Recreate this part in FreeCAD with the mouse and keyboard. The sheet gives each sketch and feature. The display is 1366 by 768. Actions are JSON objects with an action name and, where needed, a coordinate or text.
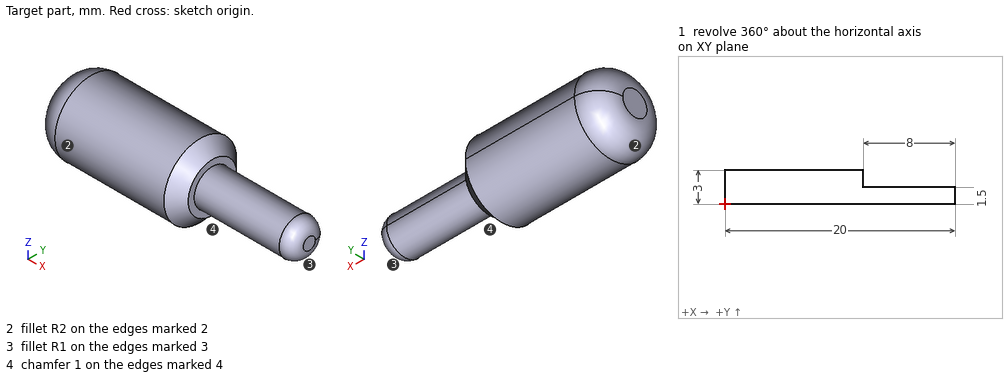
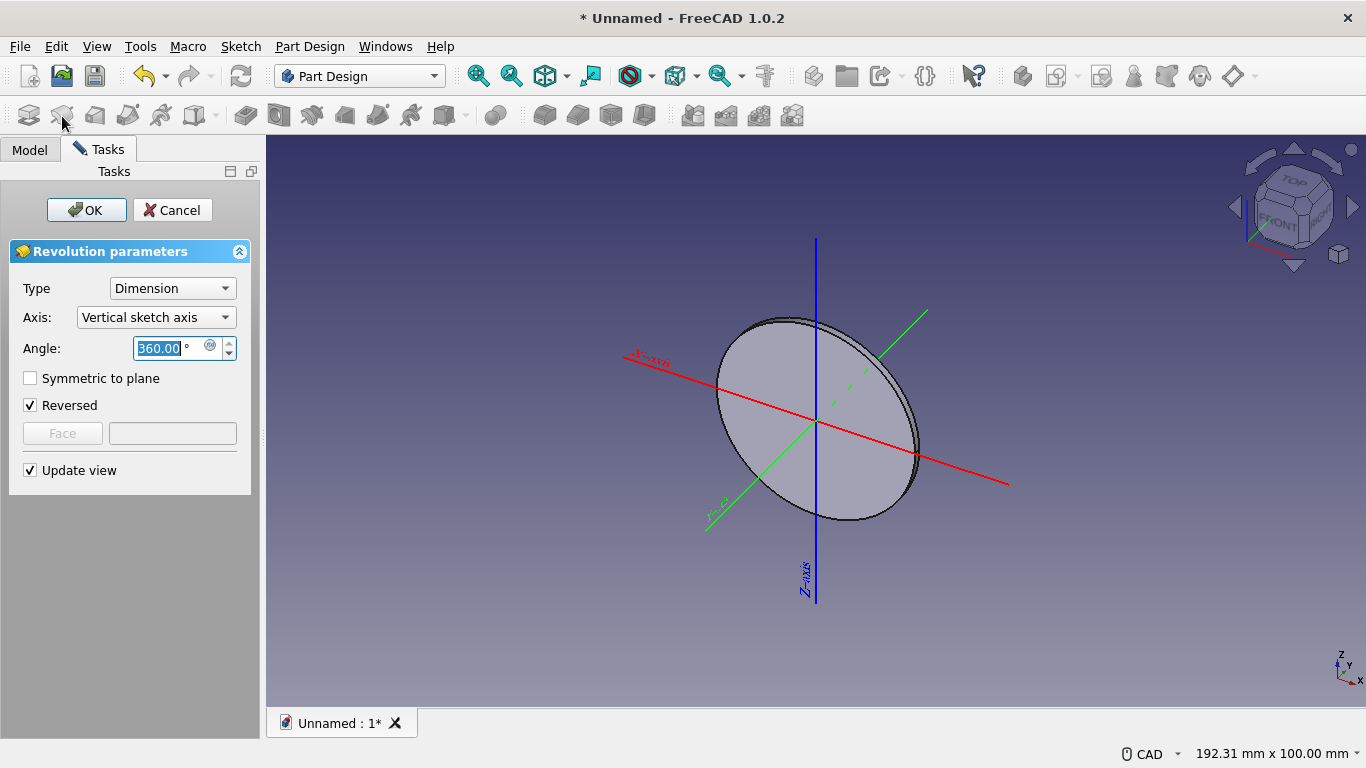
{"action": "left_click", "coordinate": [157, 318]}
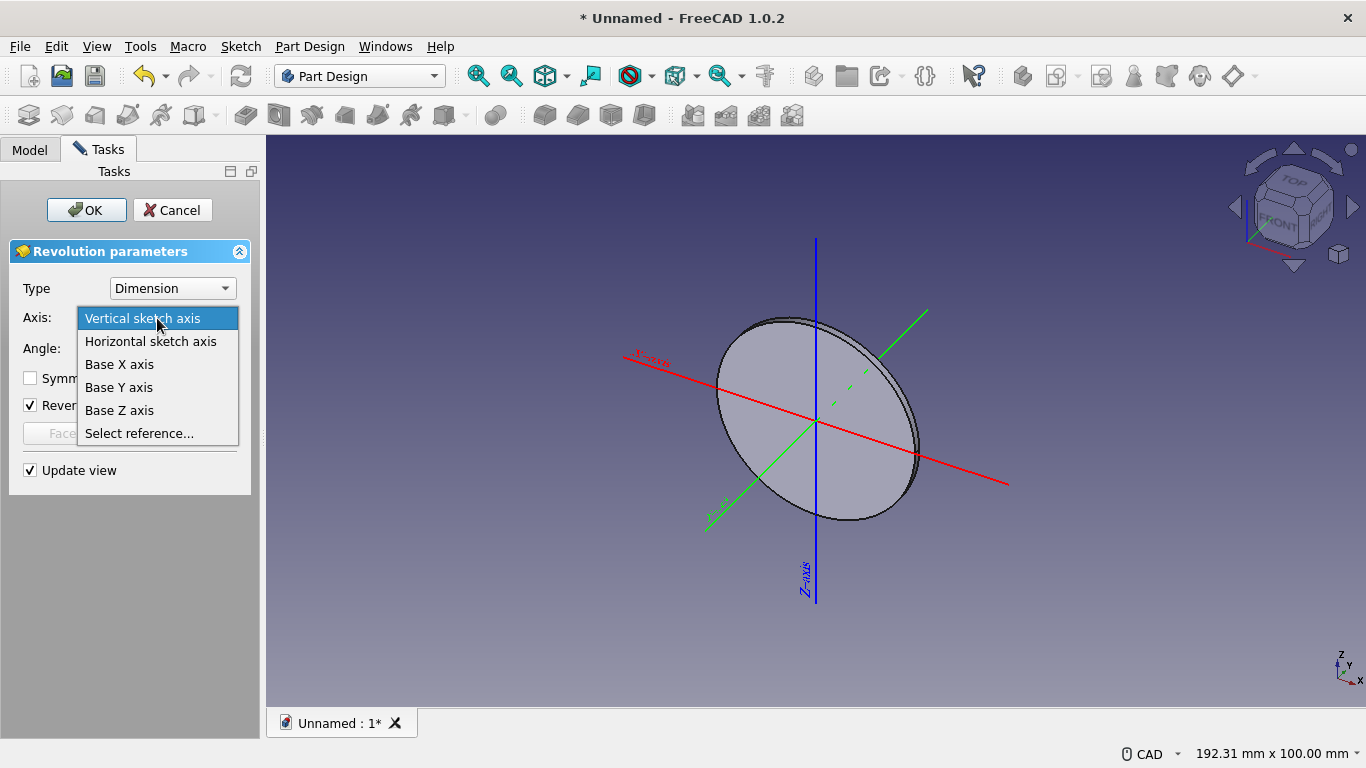
{"action": "left_click", "coordinate": [156, 342]}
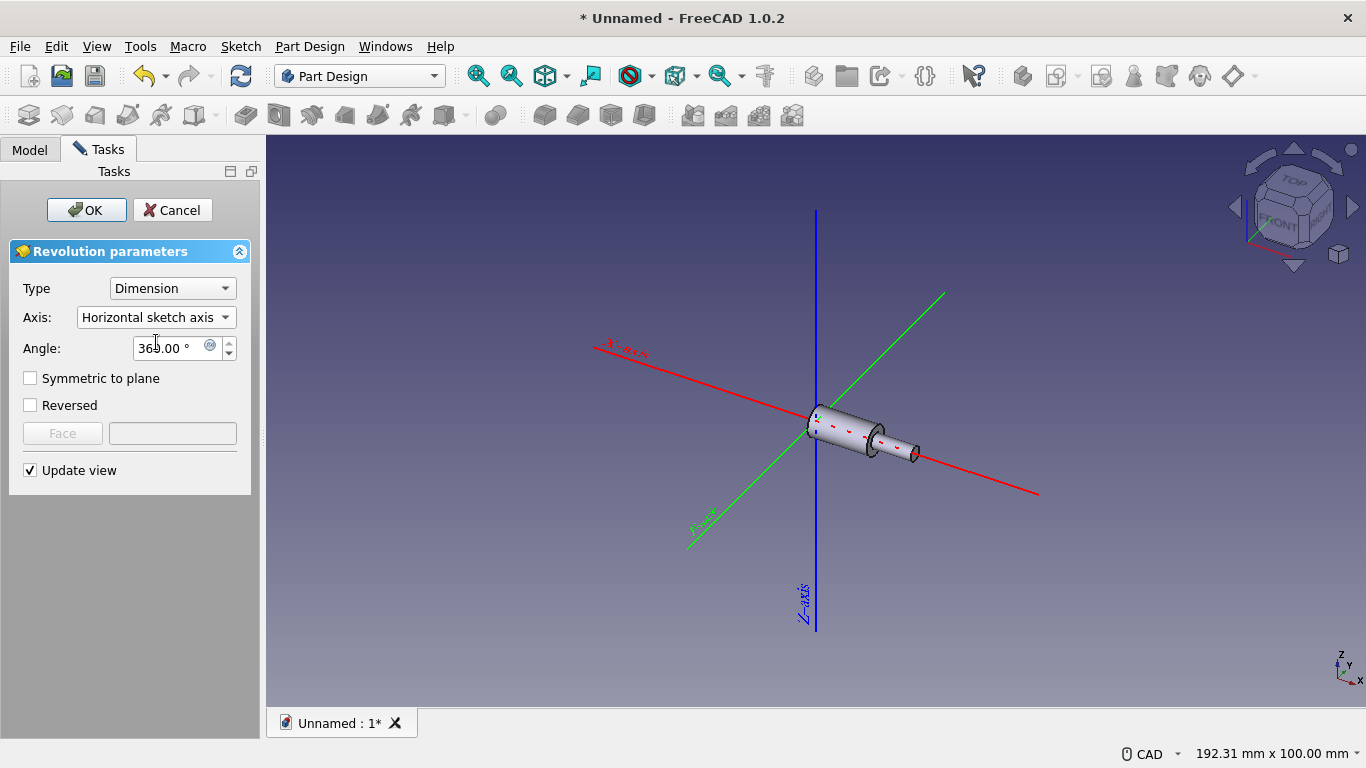
{"action": "left_click", "coordinate": [87, 210]}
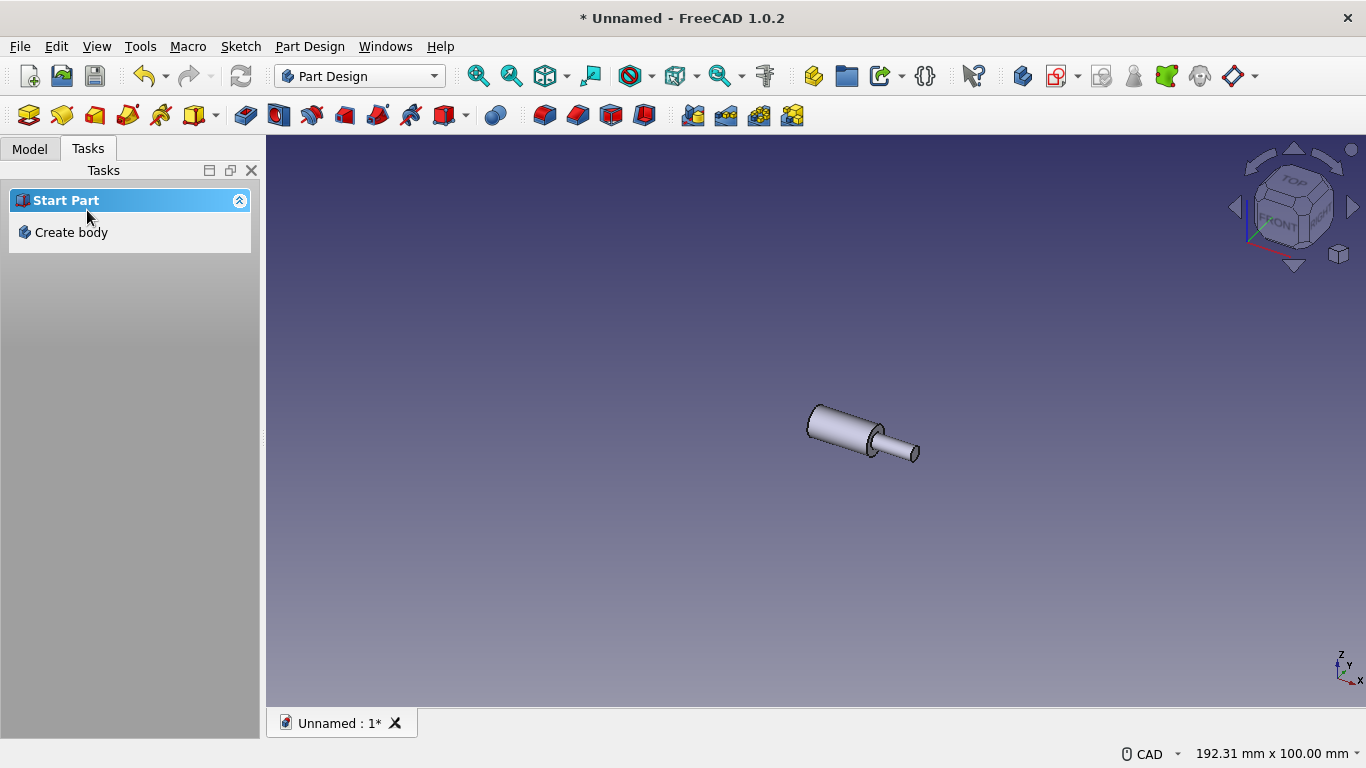
{"action": "left_click", "coordinate": [479, 76]}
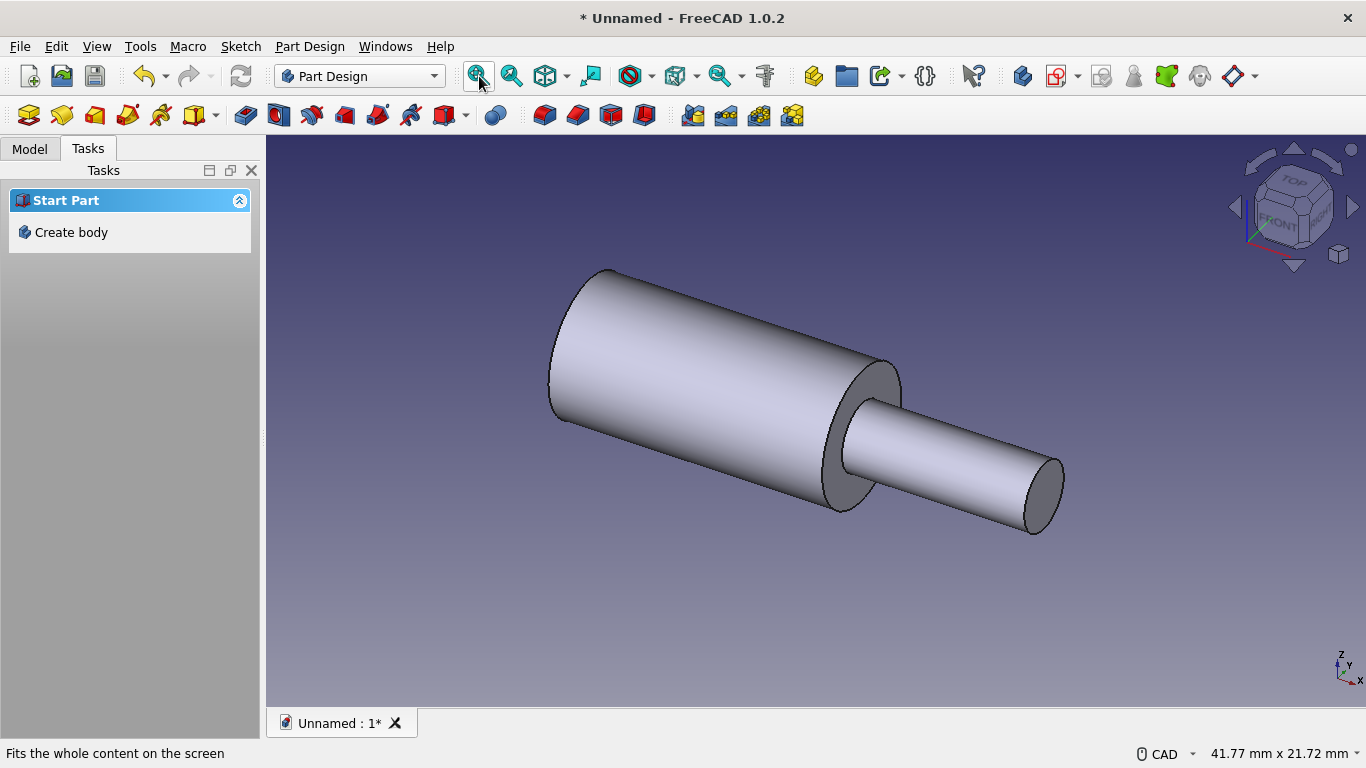
{"action": "left_click", "coordinate": [600, 271]}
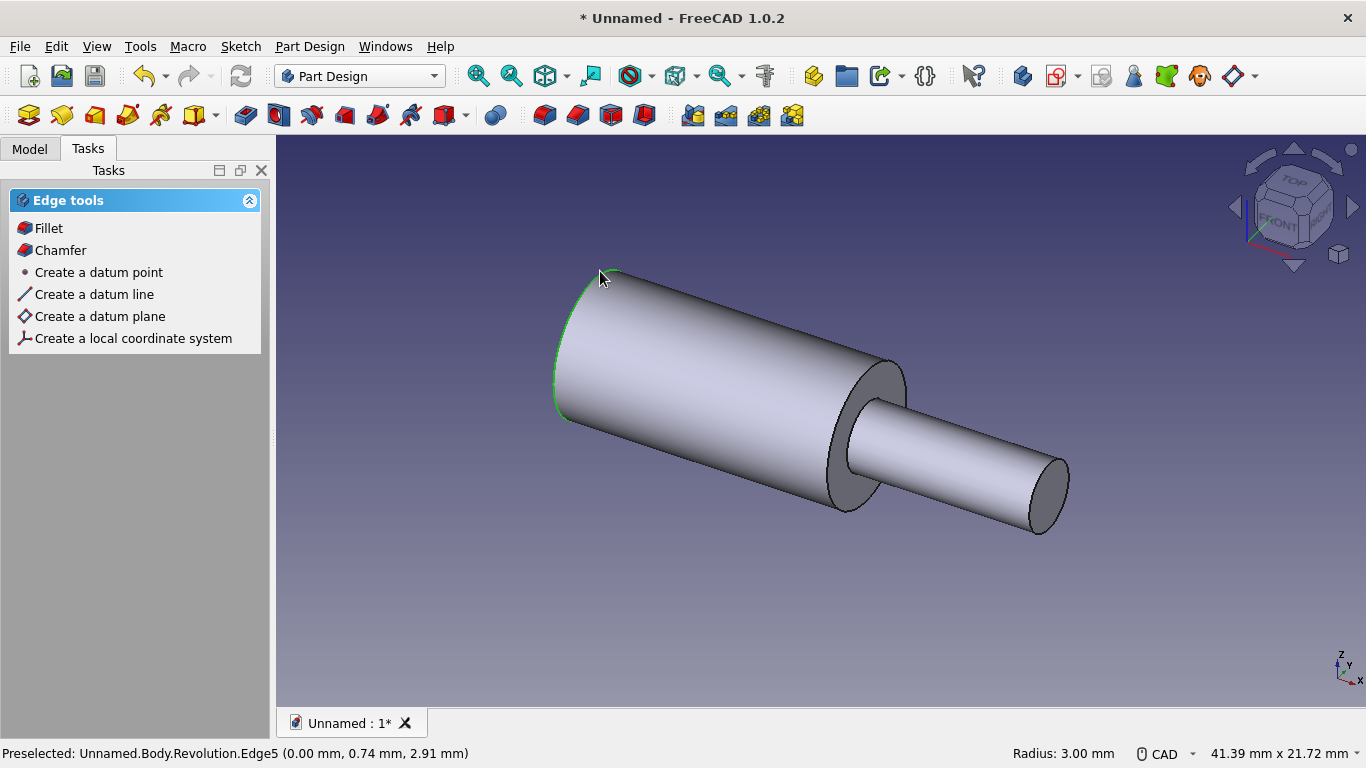
{"action": "left_click", "coordinate": [545, 116]}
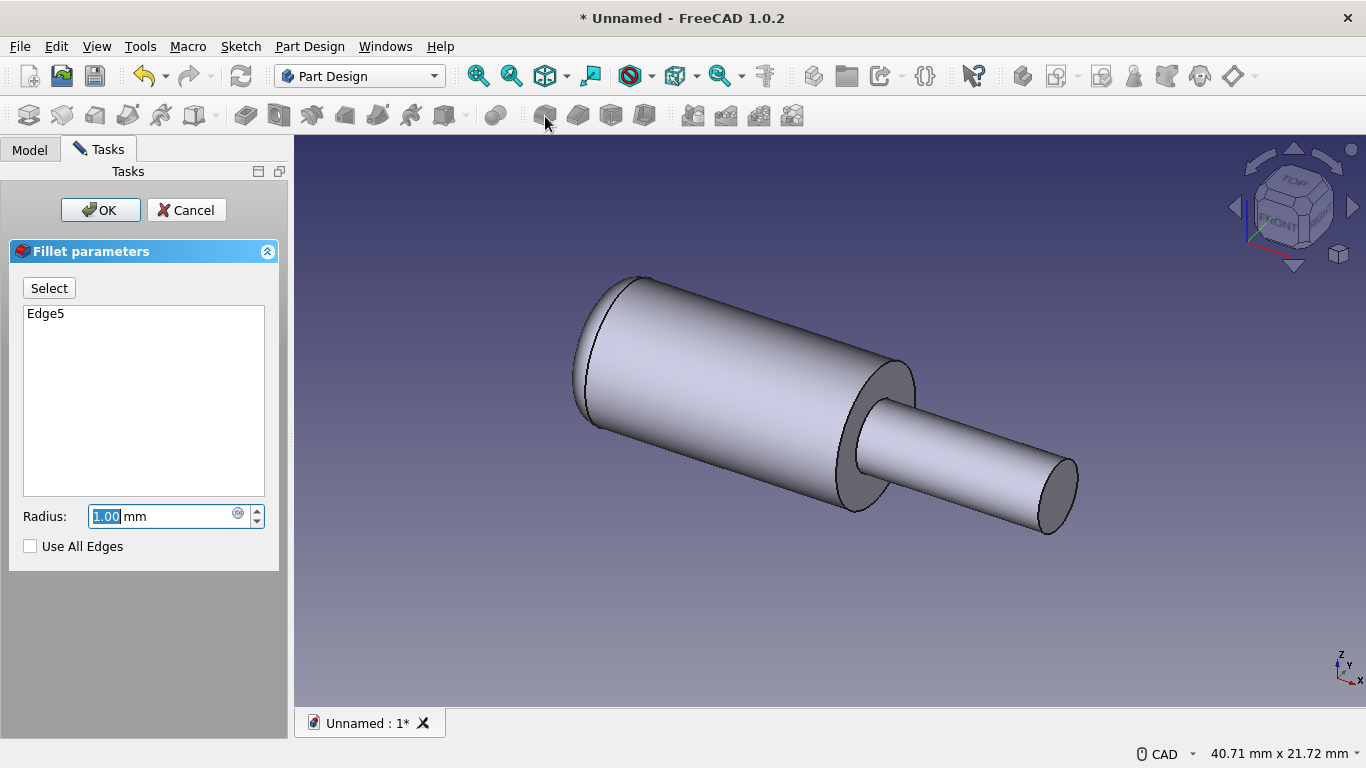
{"action": "type", "text": "2"}
{"action": "key", "text": "Tab"}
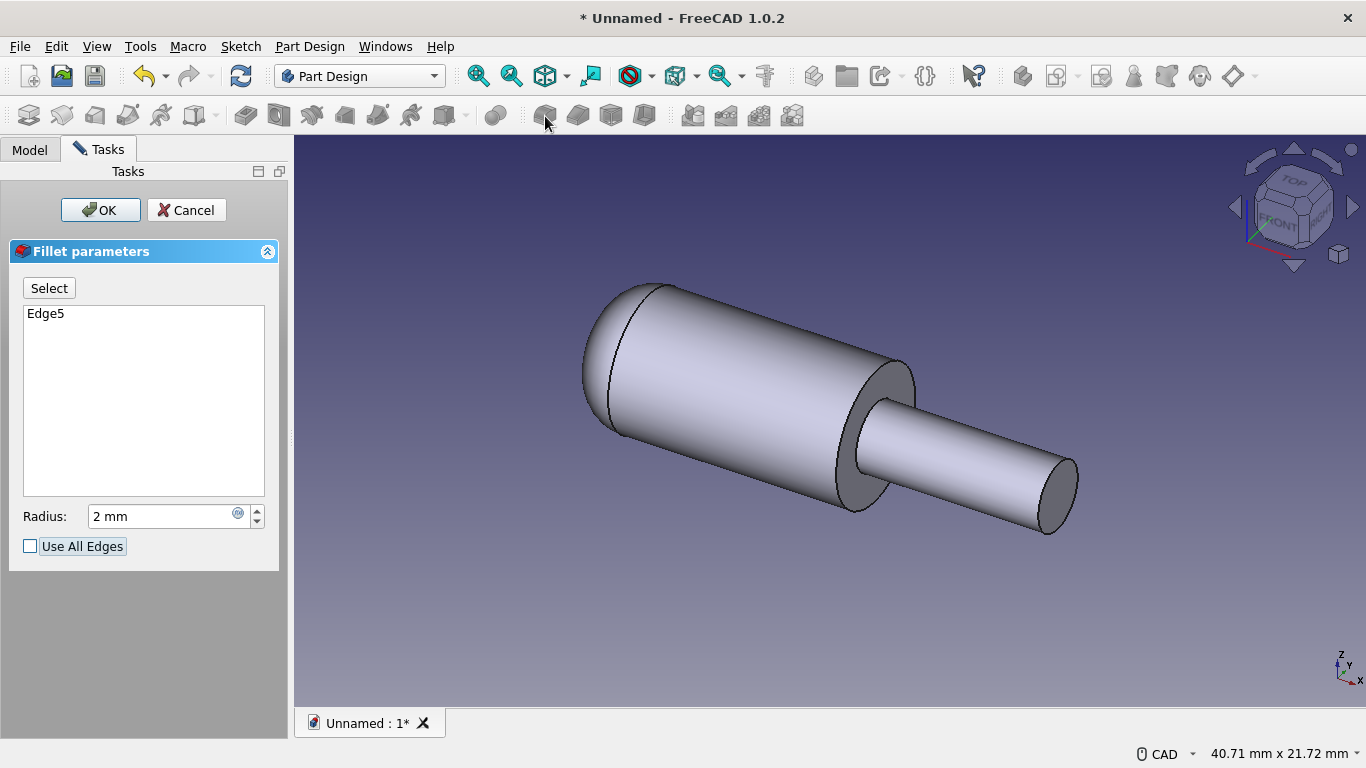
{"action": "left_click", "coordinate": [101, 210]}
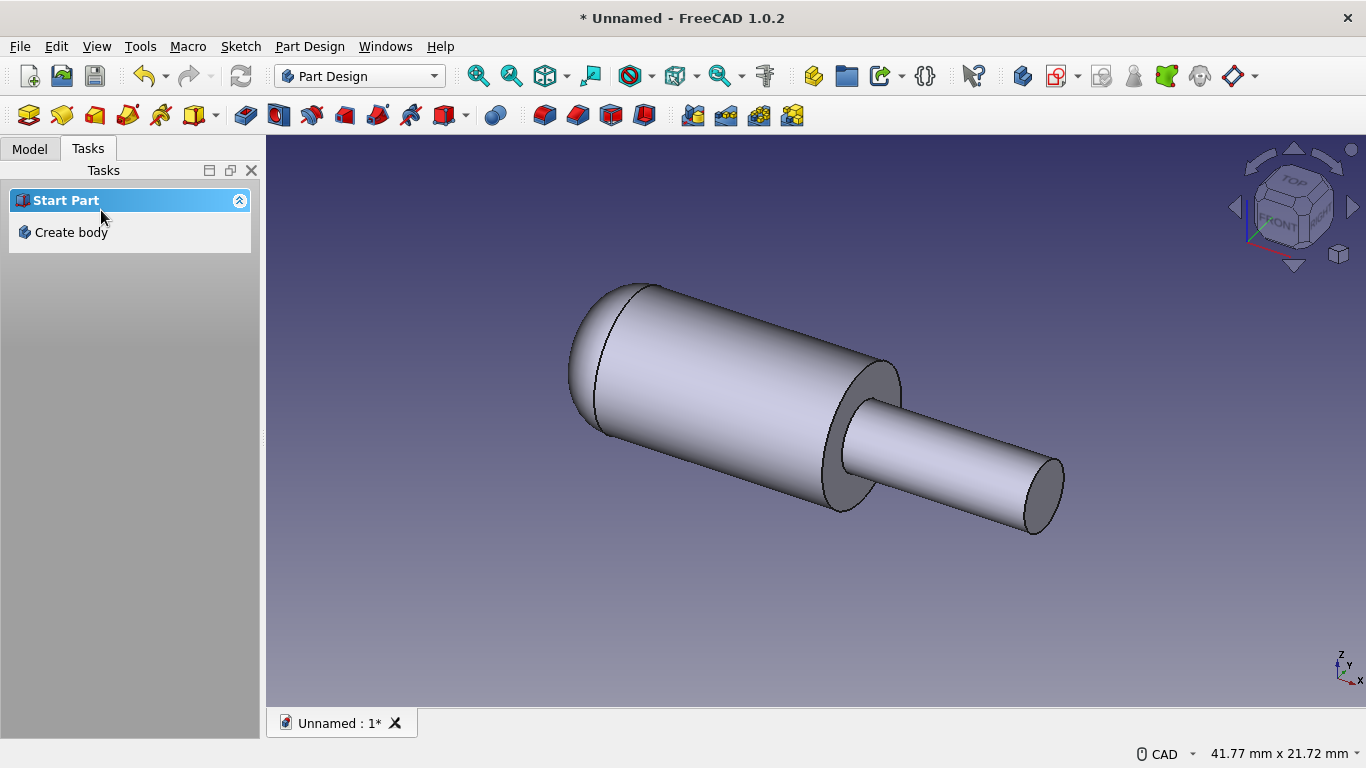
{"action": "left_click", "coordinate": [1024, 515]}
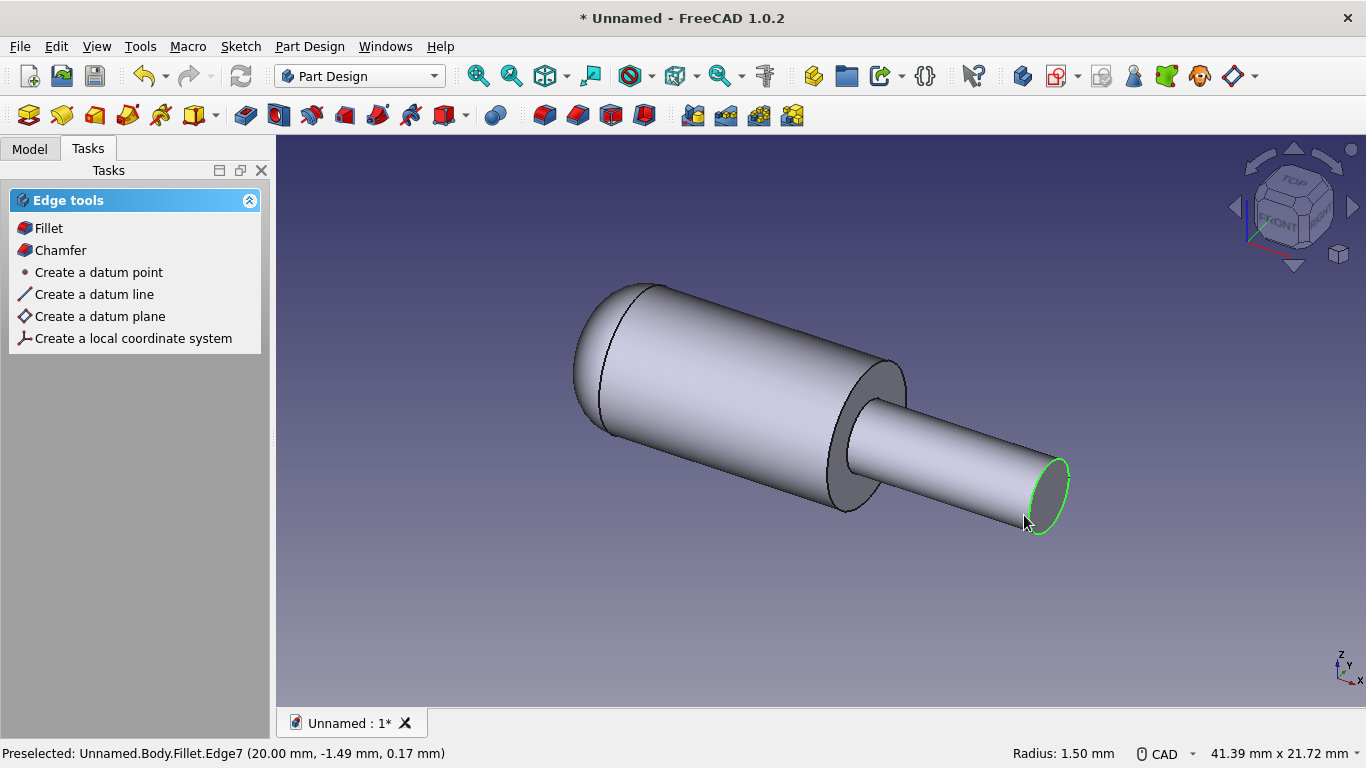
{"action": "left_click", "coordinate": [545, 116]}